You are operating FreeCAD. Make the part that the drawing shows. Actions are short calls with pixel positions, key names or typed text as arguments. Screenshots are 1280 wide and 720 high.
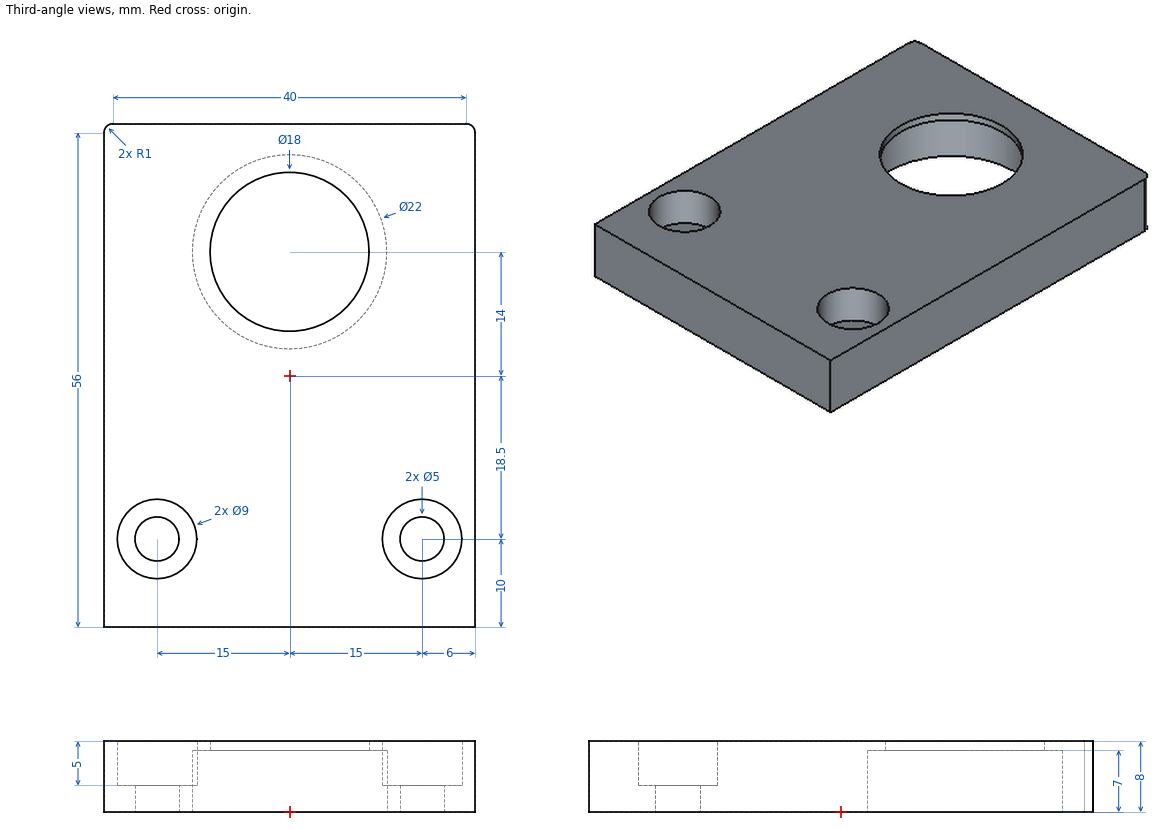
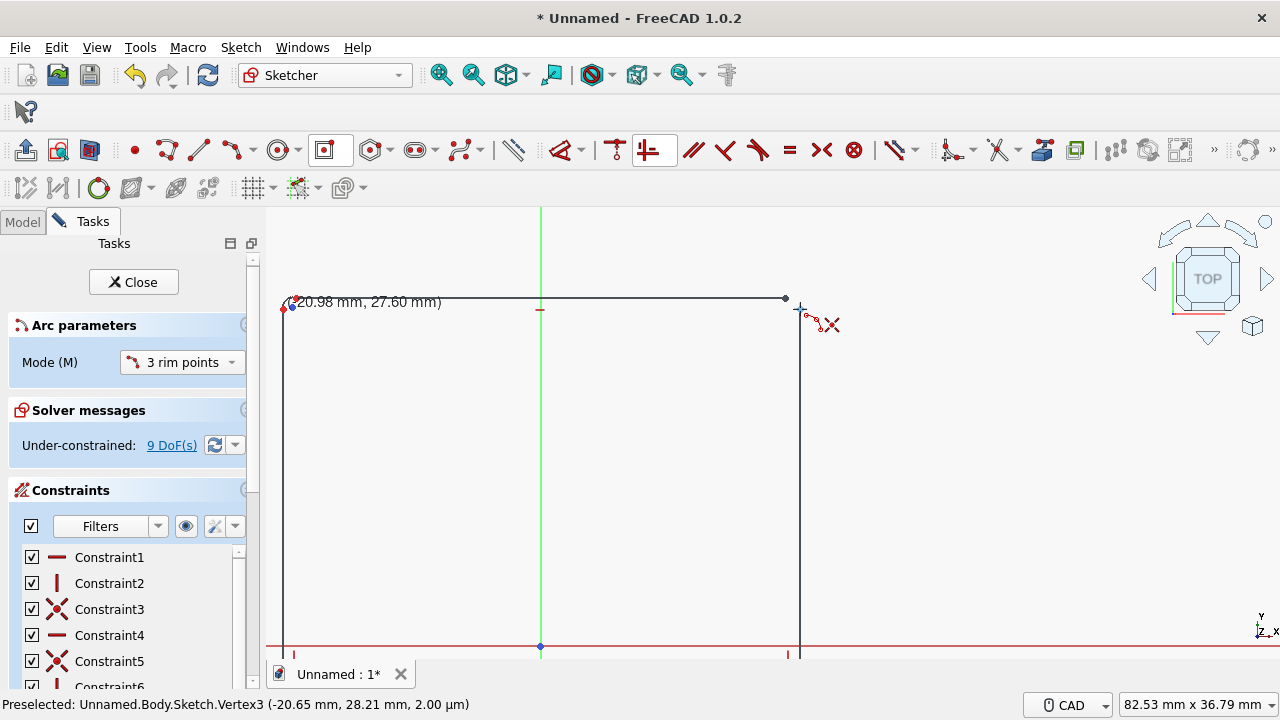
click(800, 309)
click(786, 298)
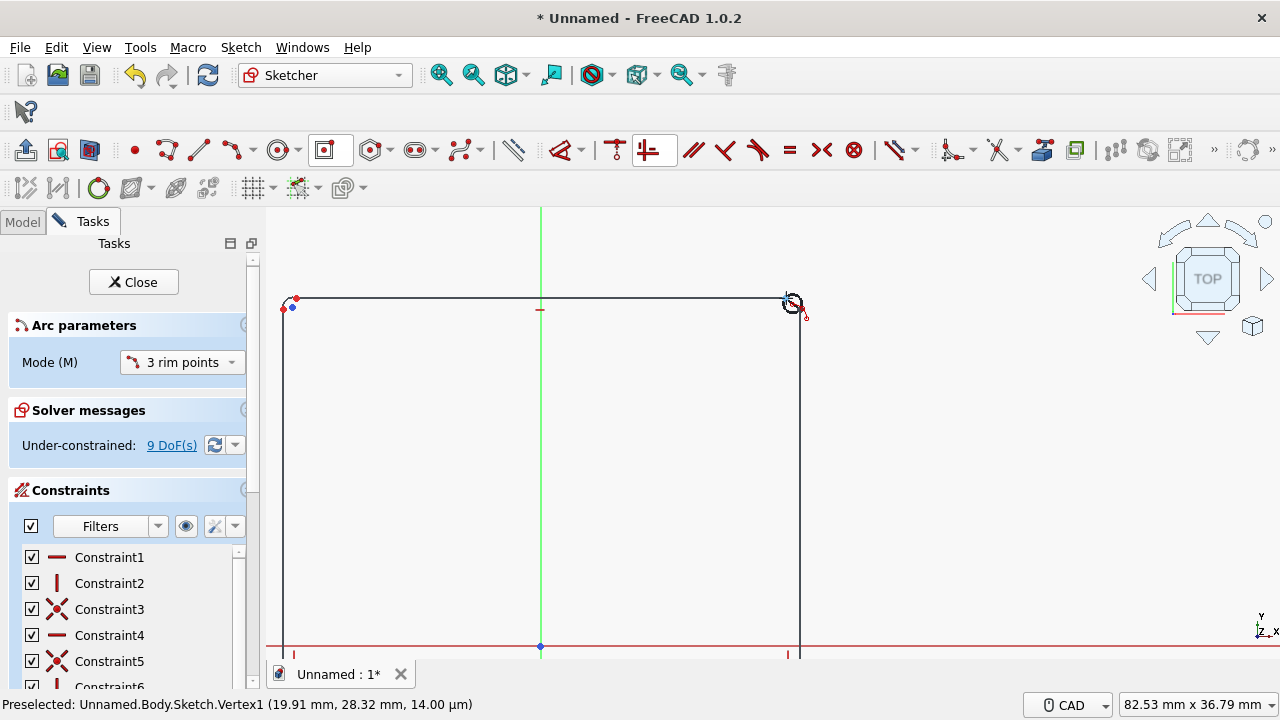
scroll(795, 300, up, 8)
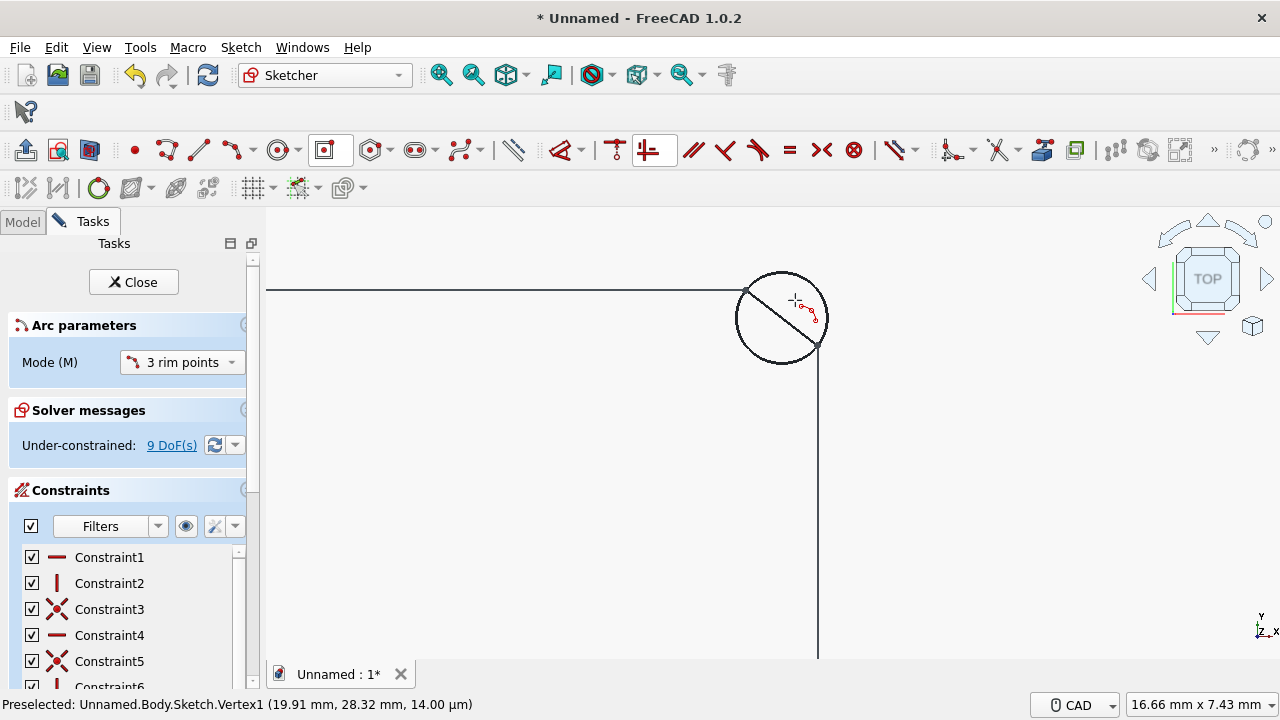
click(794, 297)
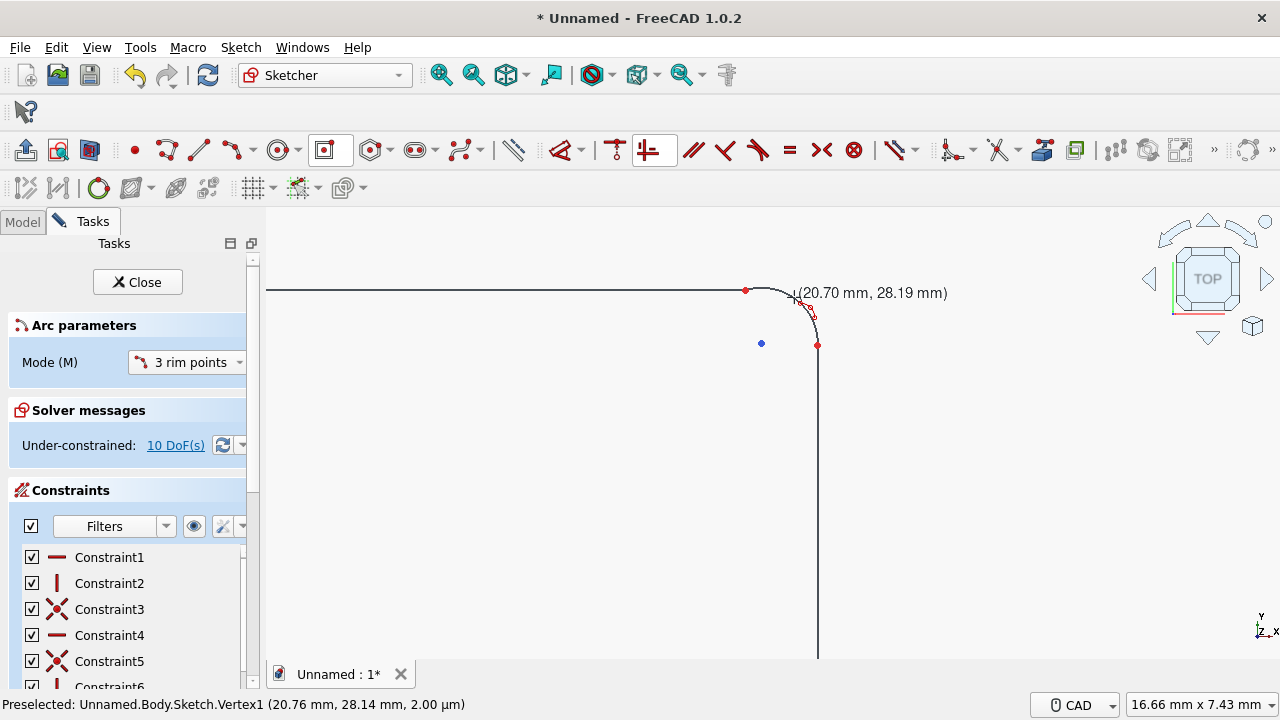
click(278, 150)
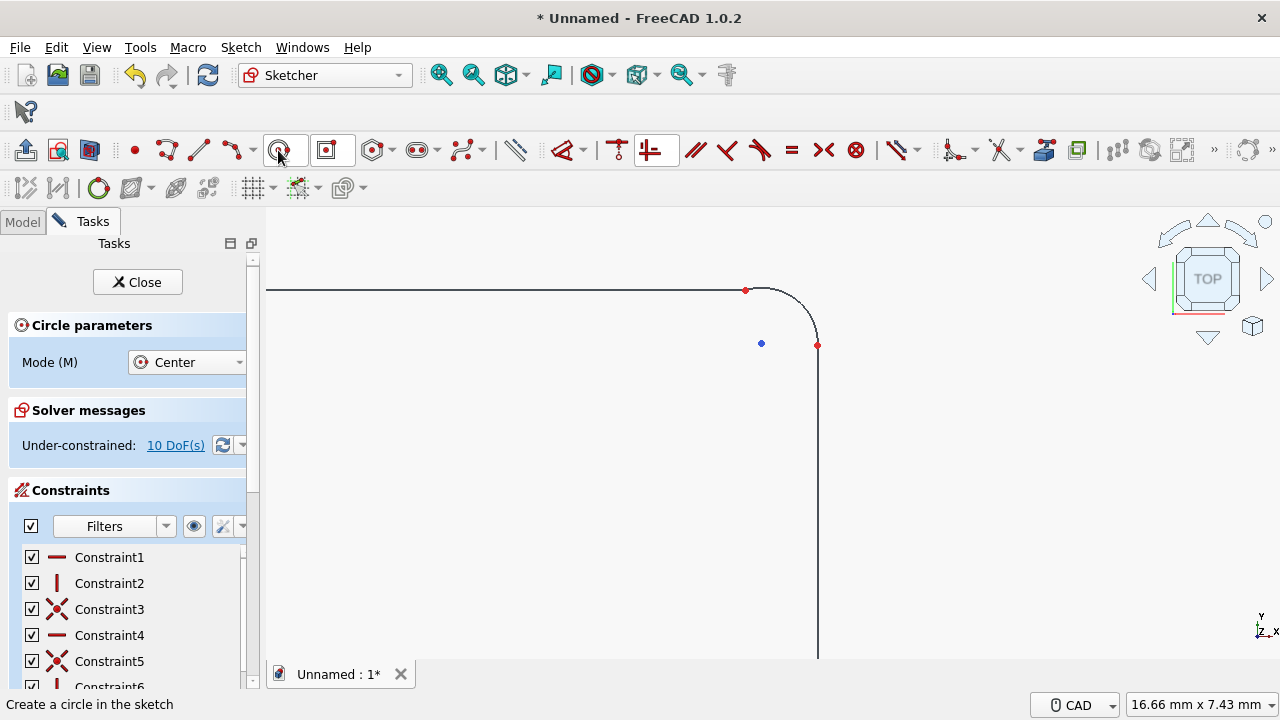
scroll(798, 306, down, 13)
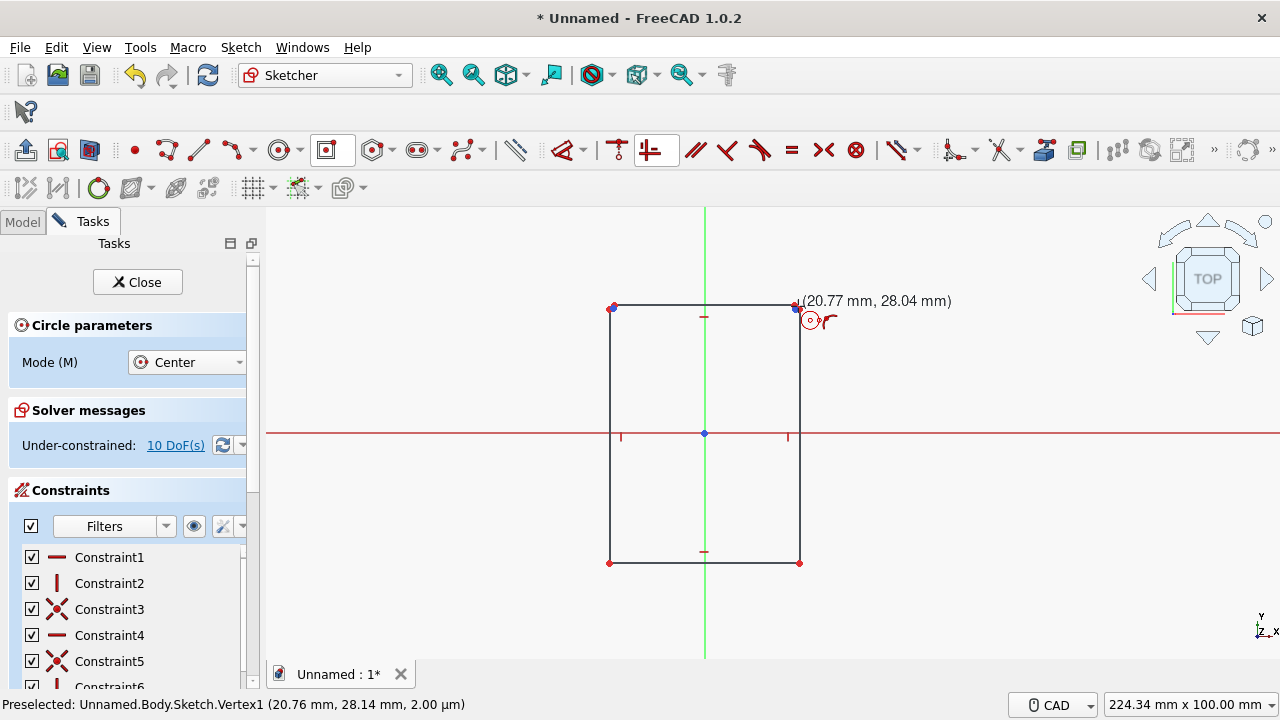
scroll(772, 517, up, 4)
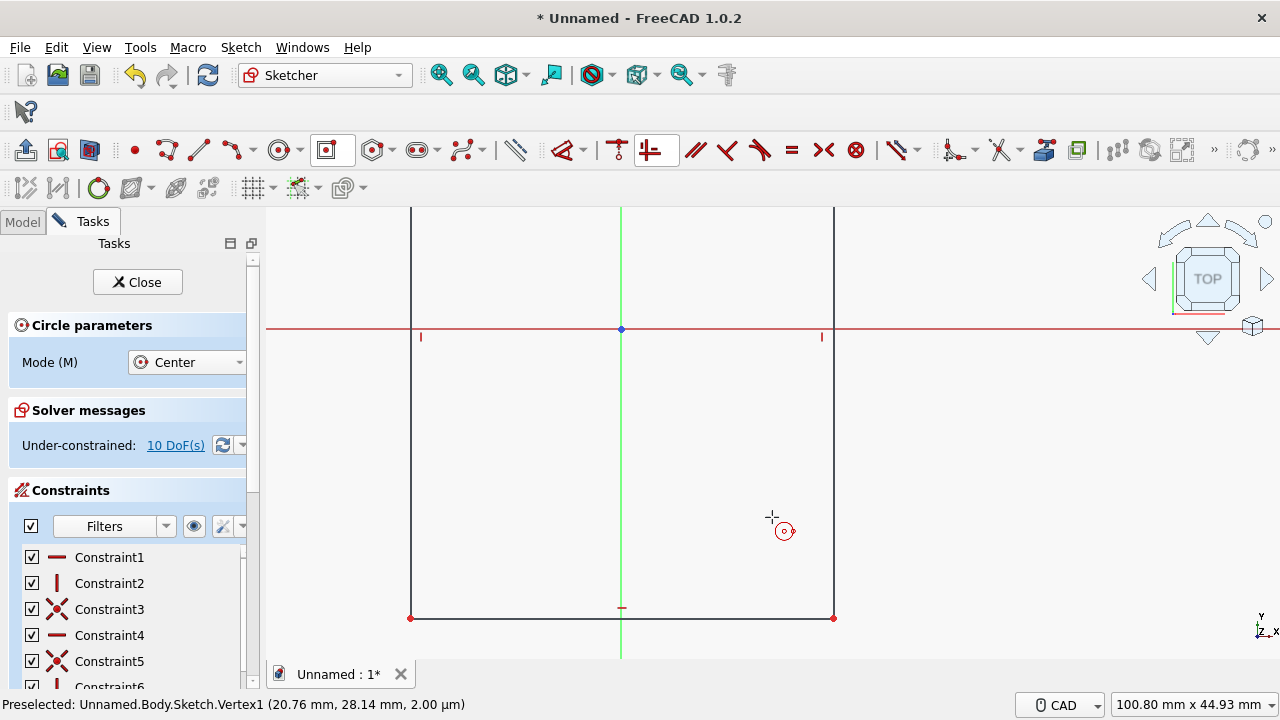
click(772, 515)
click(790, 498)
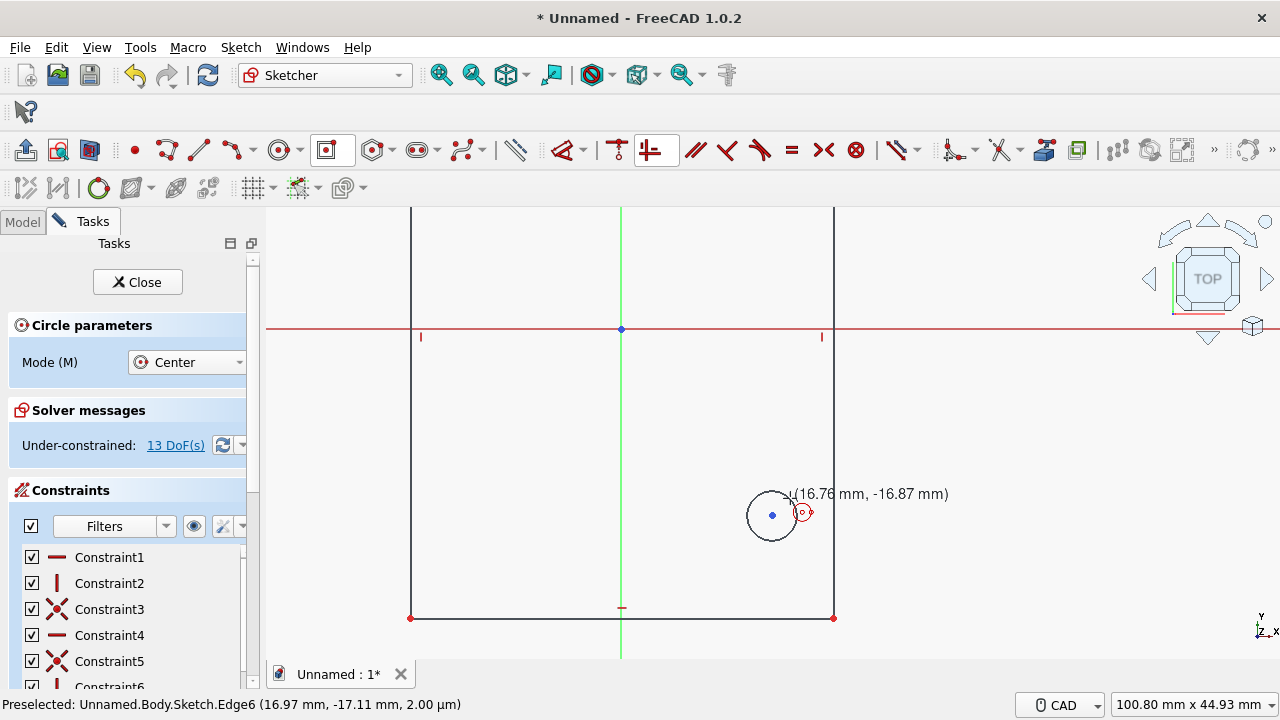
click(471, 515)
click(488, 498)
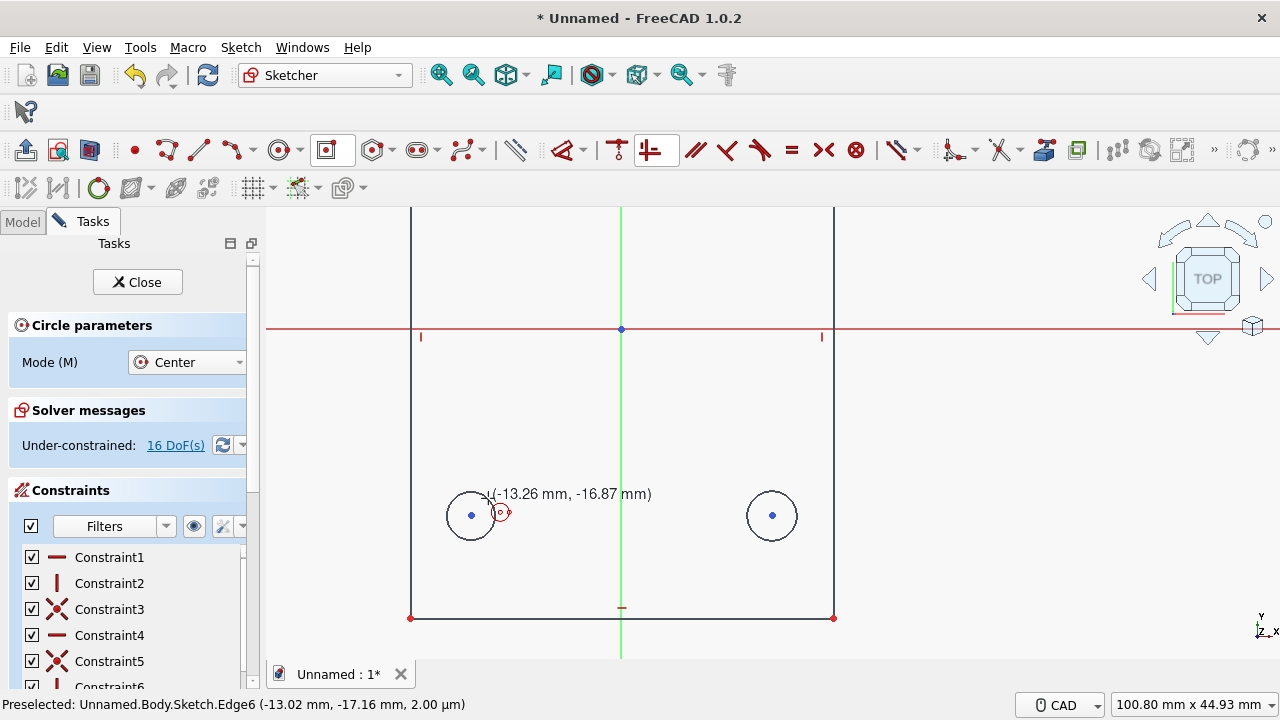
scroll(772, 518, down, 4)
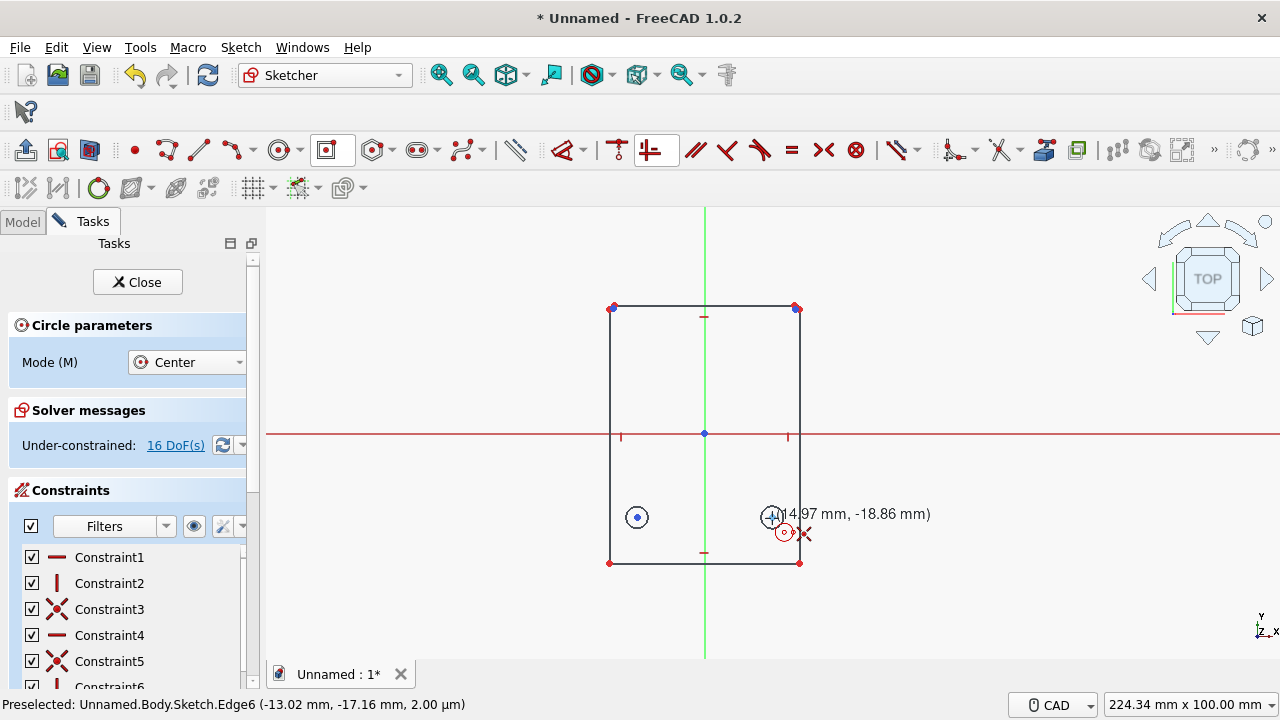
click(705, 370)
click(733, 342)
key(Escape)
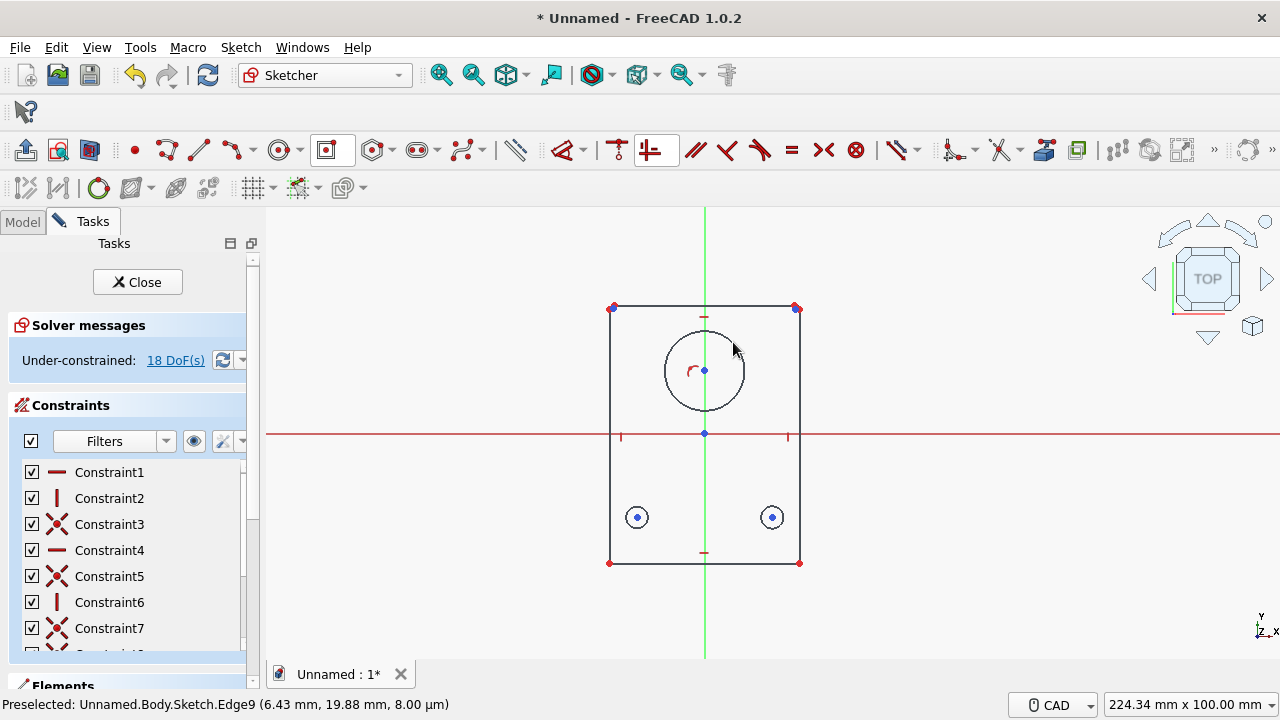
click(741, 306)